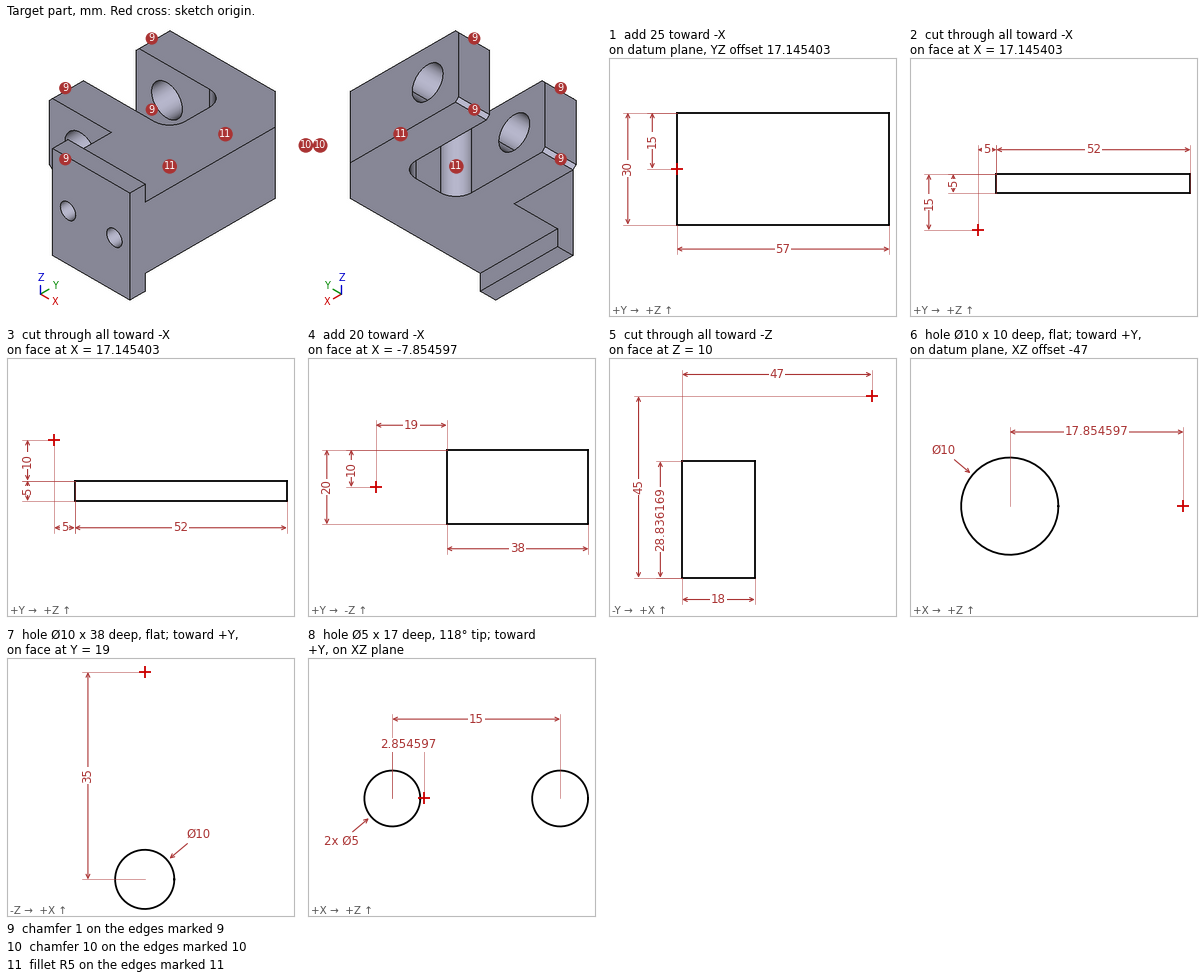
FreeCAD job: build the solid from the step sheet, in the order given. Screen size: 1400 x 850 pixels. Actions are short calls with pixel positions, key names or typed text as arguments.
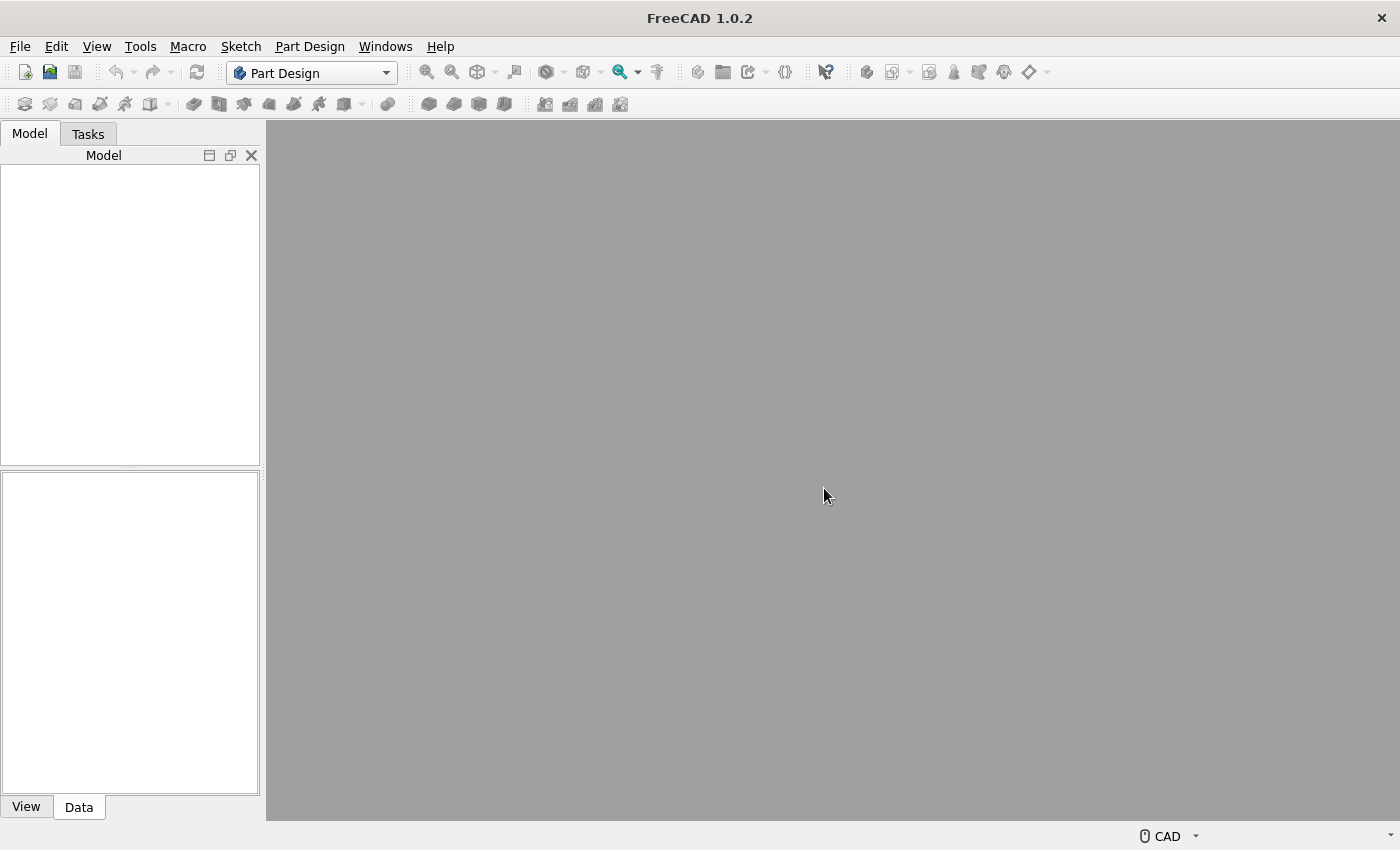
click(25, 72)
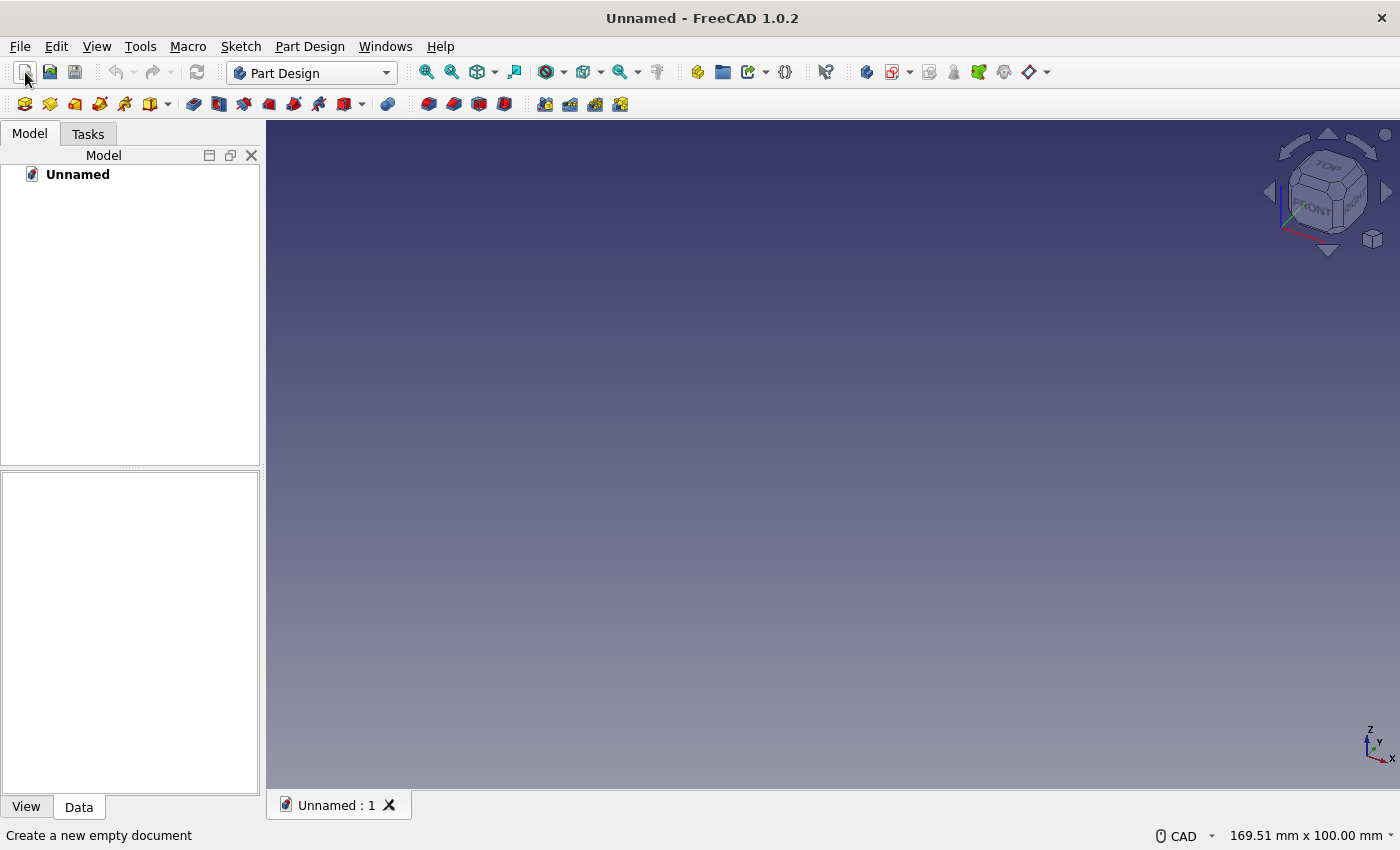
click(867, 72)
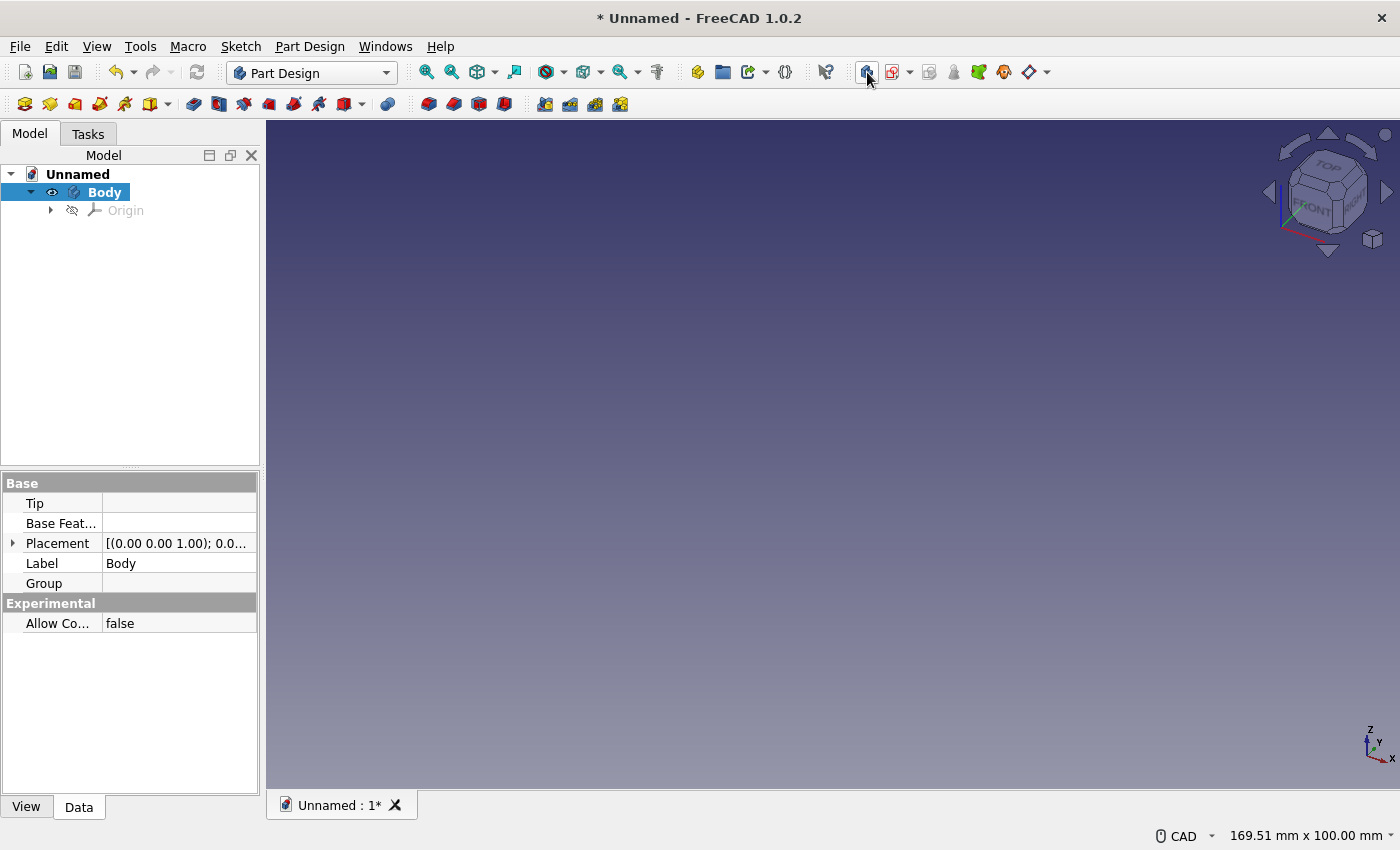
click(51, 210)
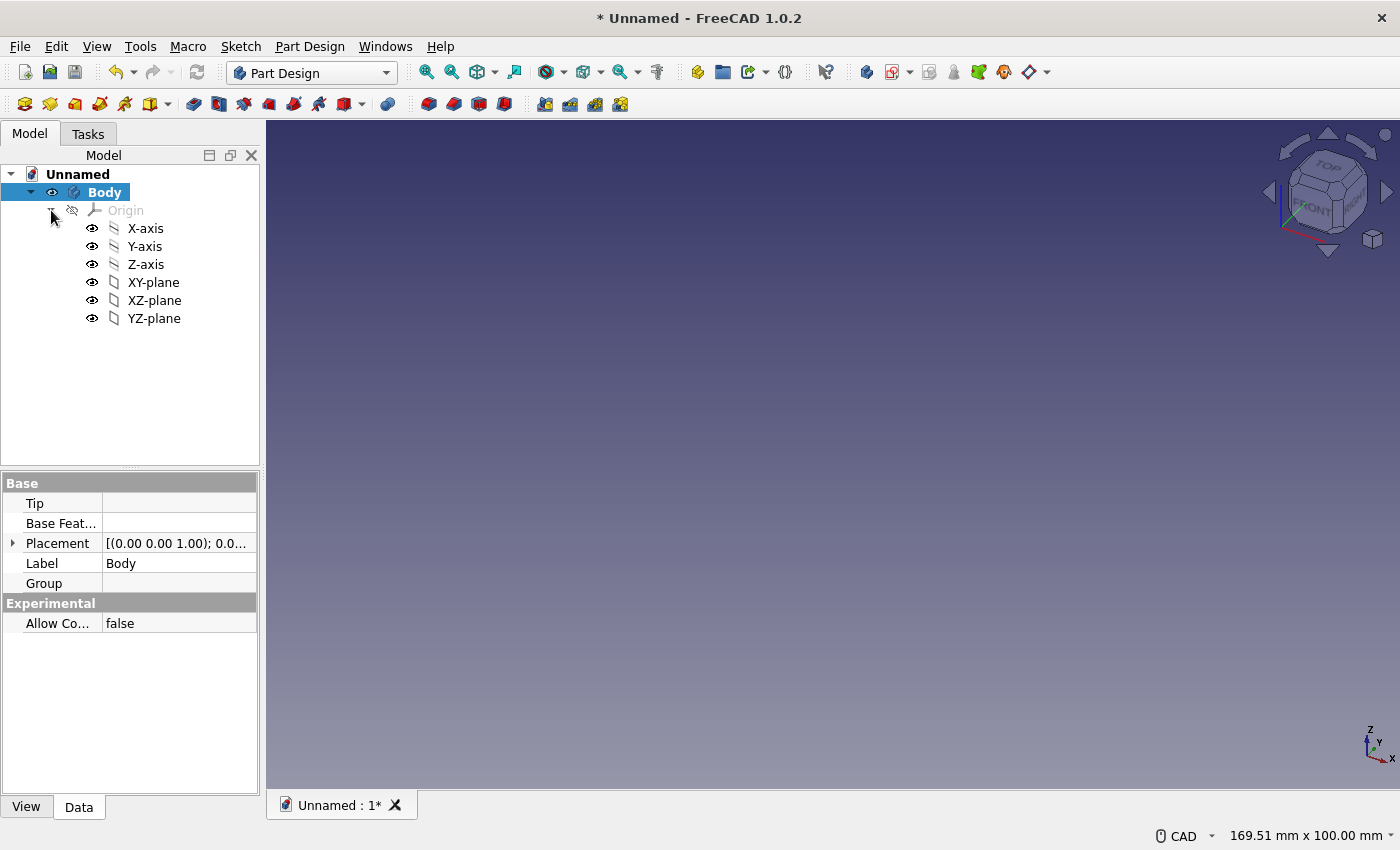
click(137, 318)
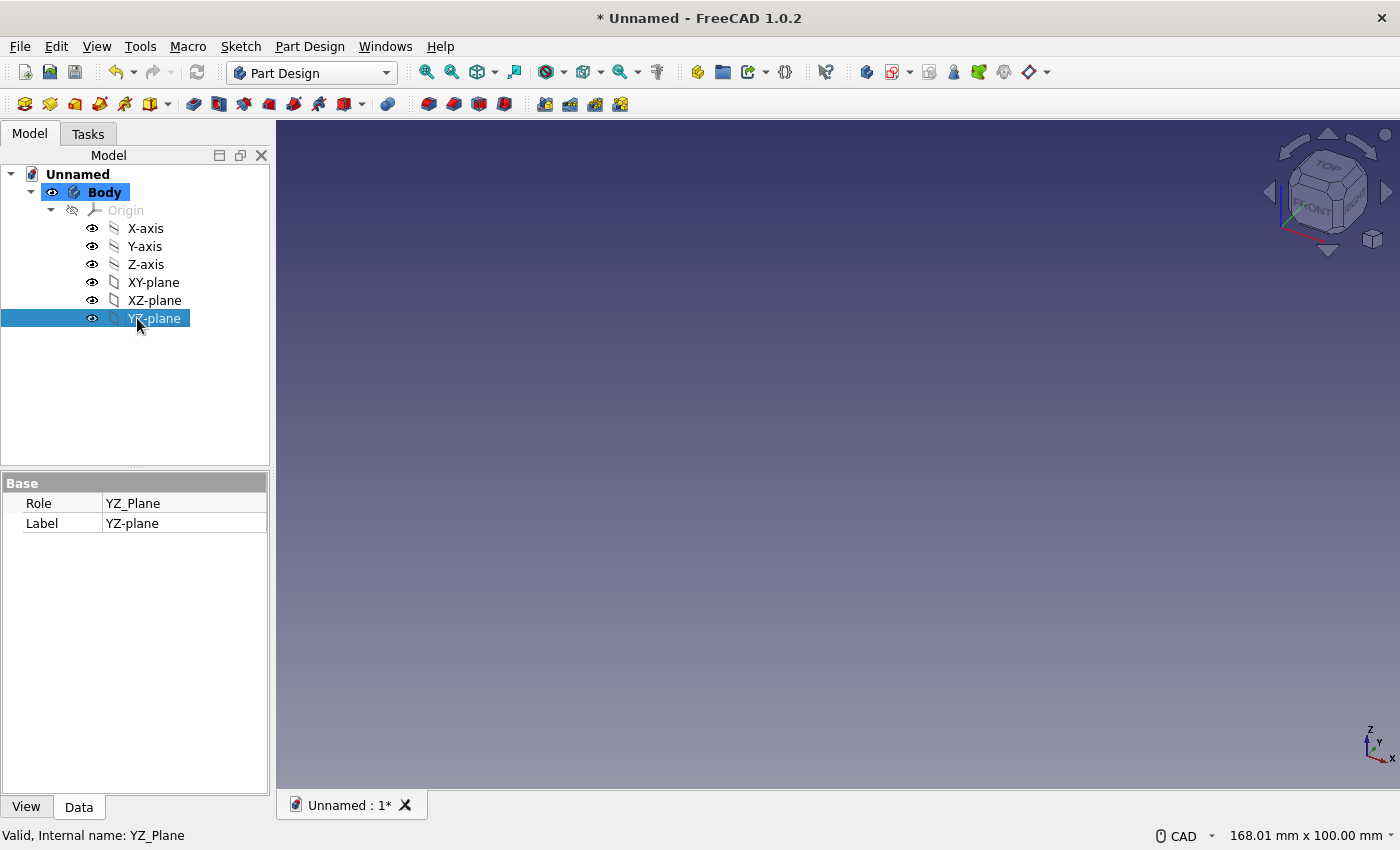
click(1028, 72)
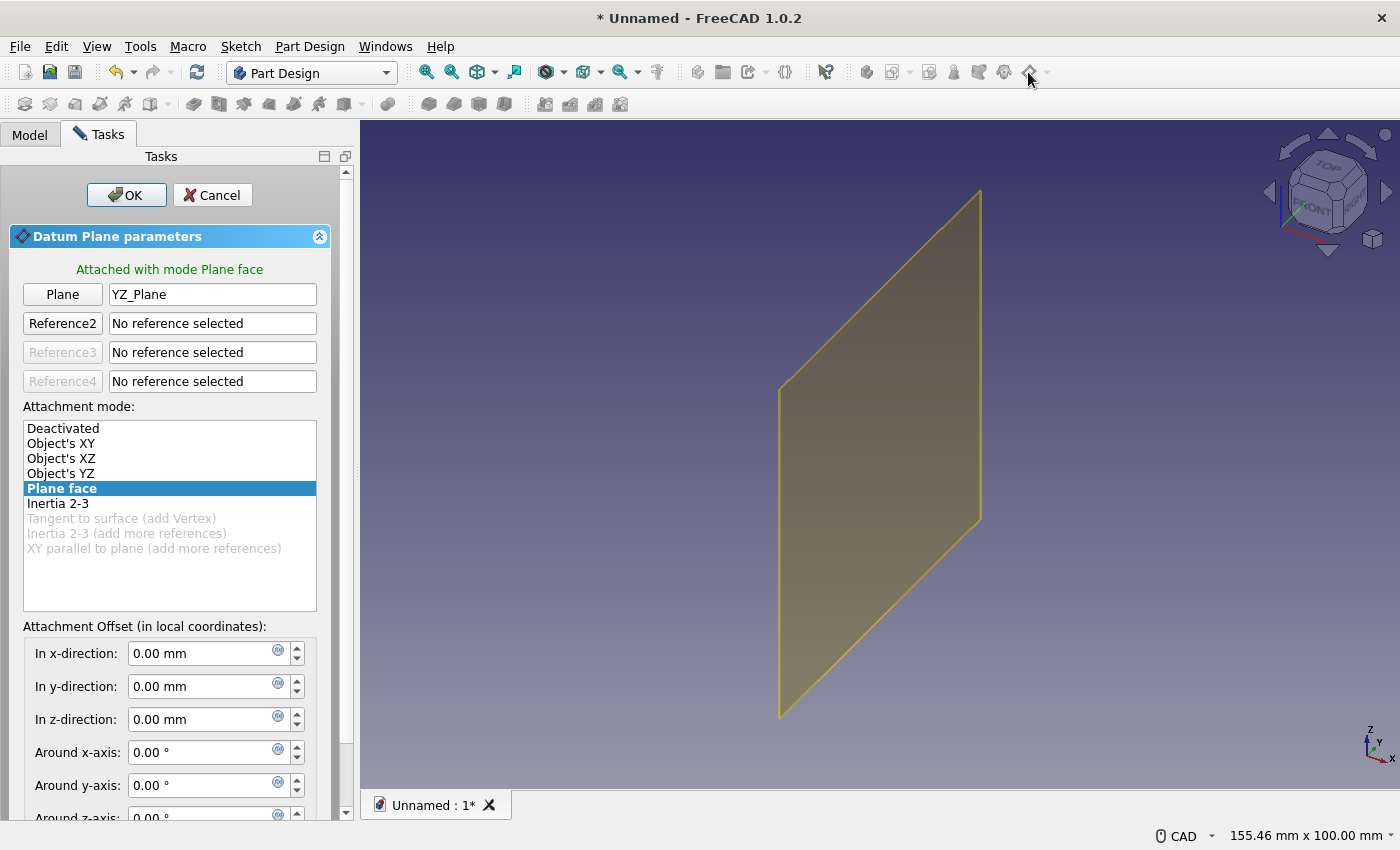
triple_click(210, 720)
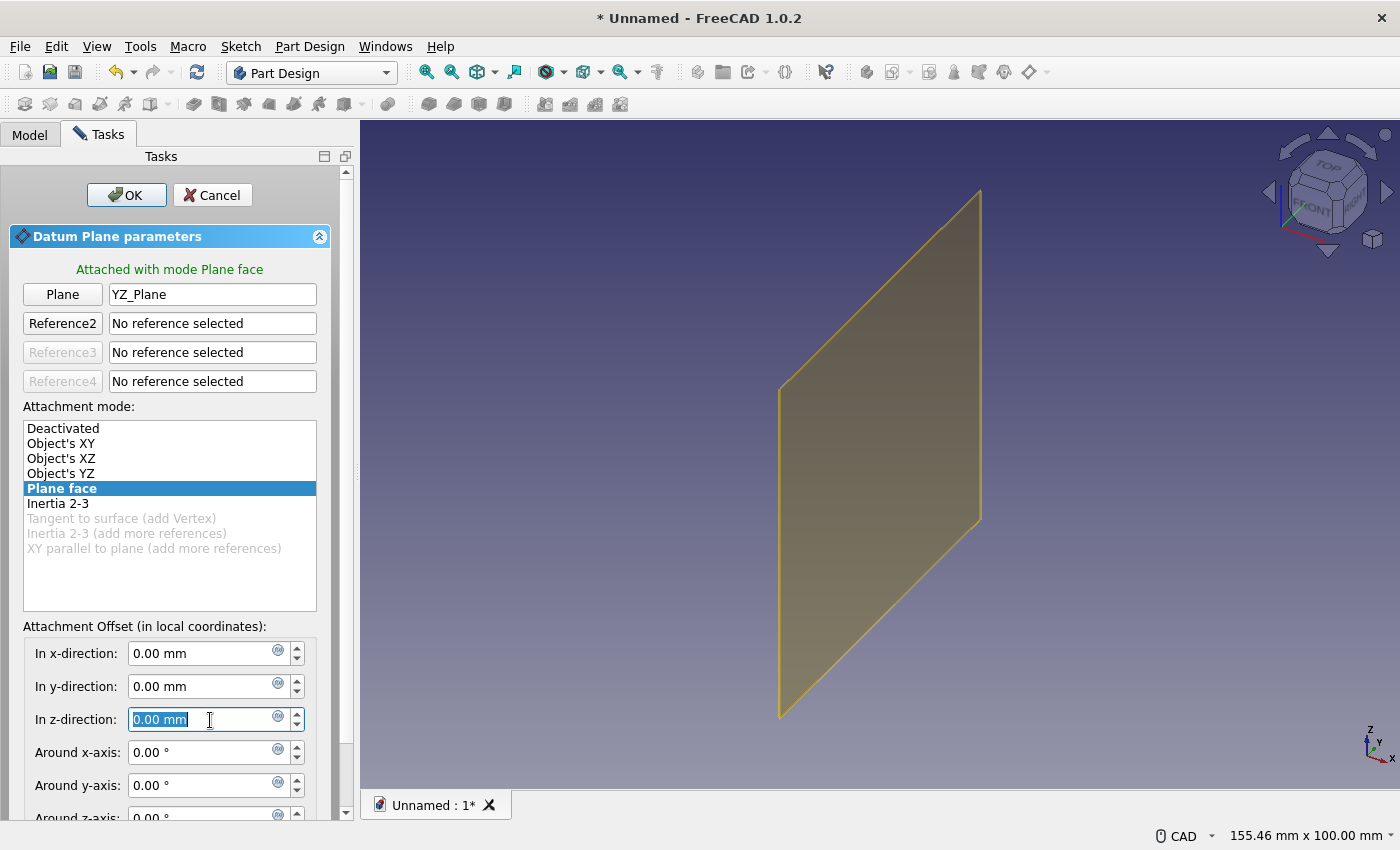
text(17.145403)
key(Tab)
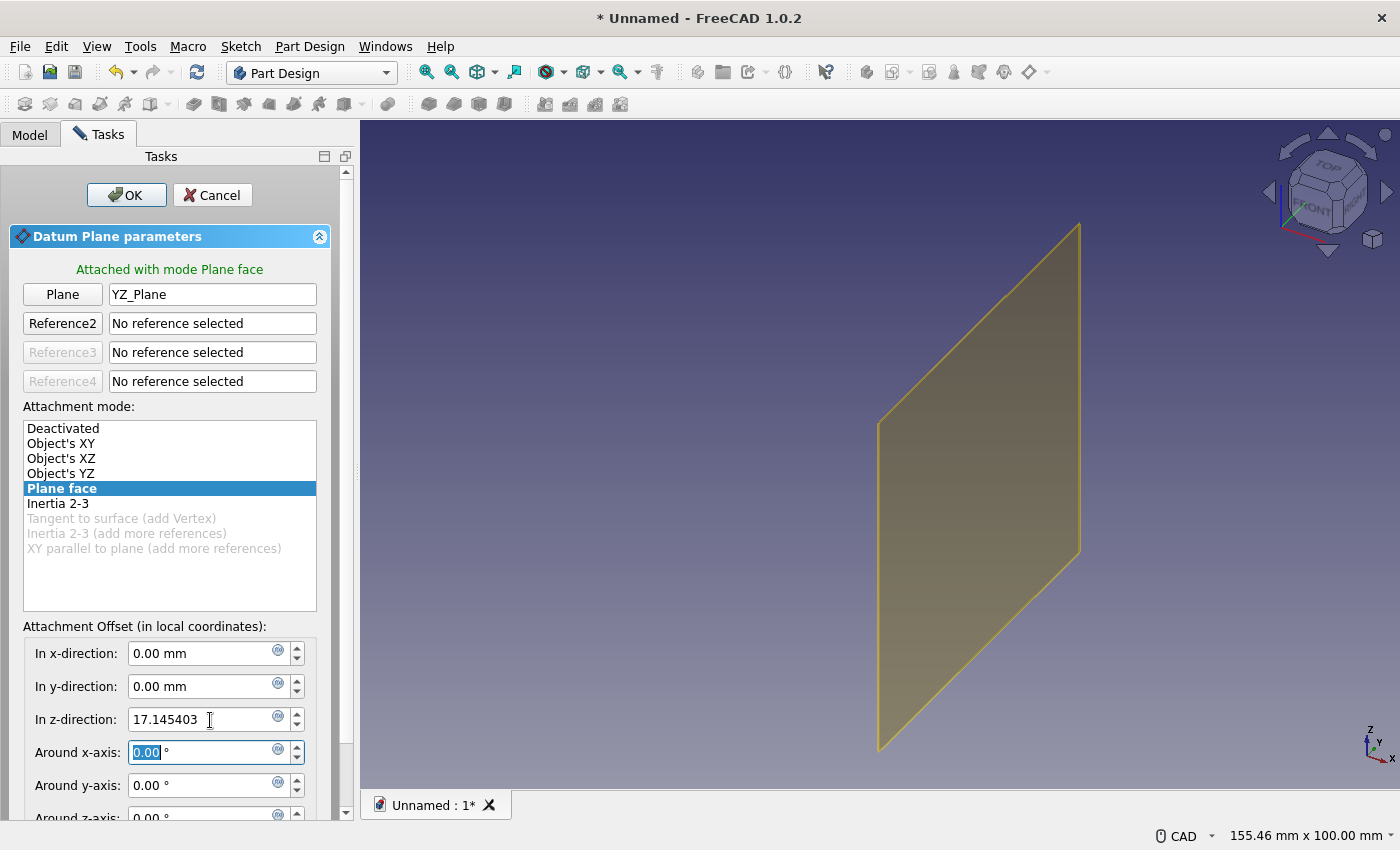
click(127, 195)